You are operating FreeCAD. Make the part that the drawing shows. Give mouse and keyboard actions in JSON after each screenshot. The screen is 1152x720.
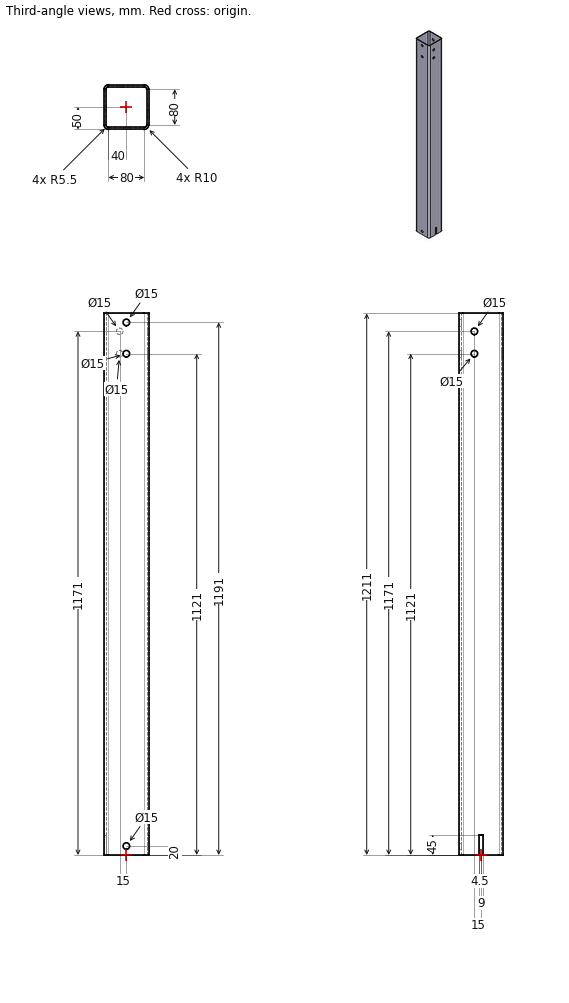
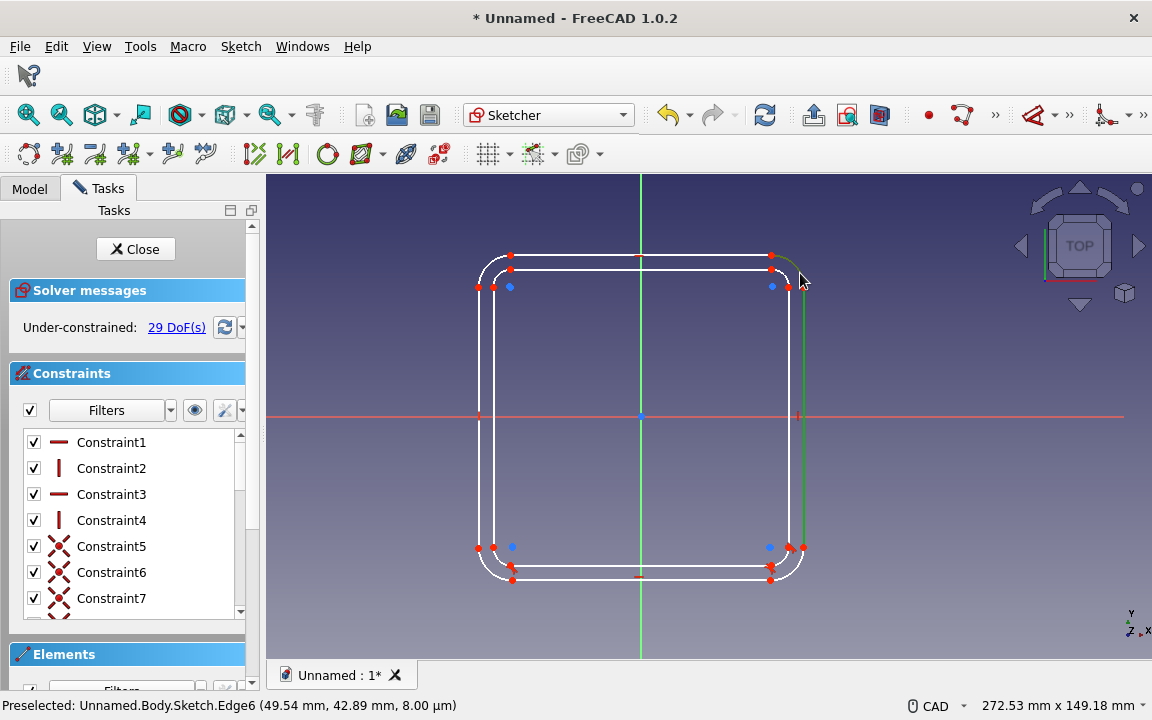
{"action": "key", "text": "t"}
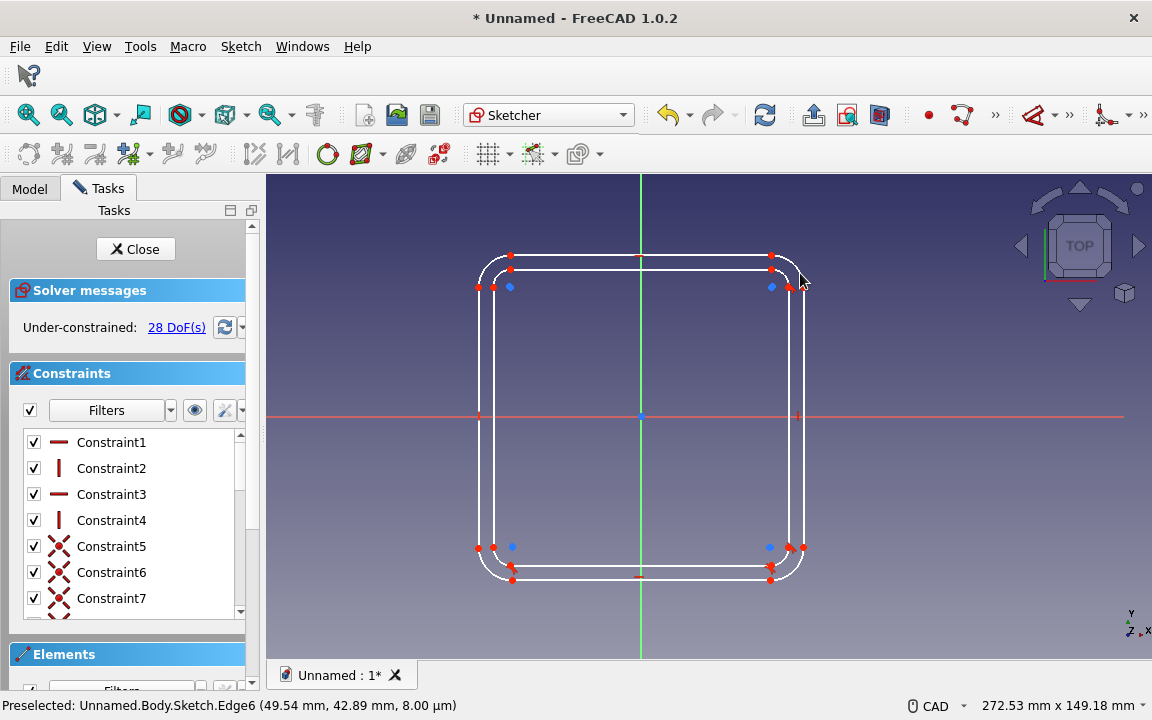
{"action": "left_click", "coordinate": [693, 255]}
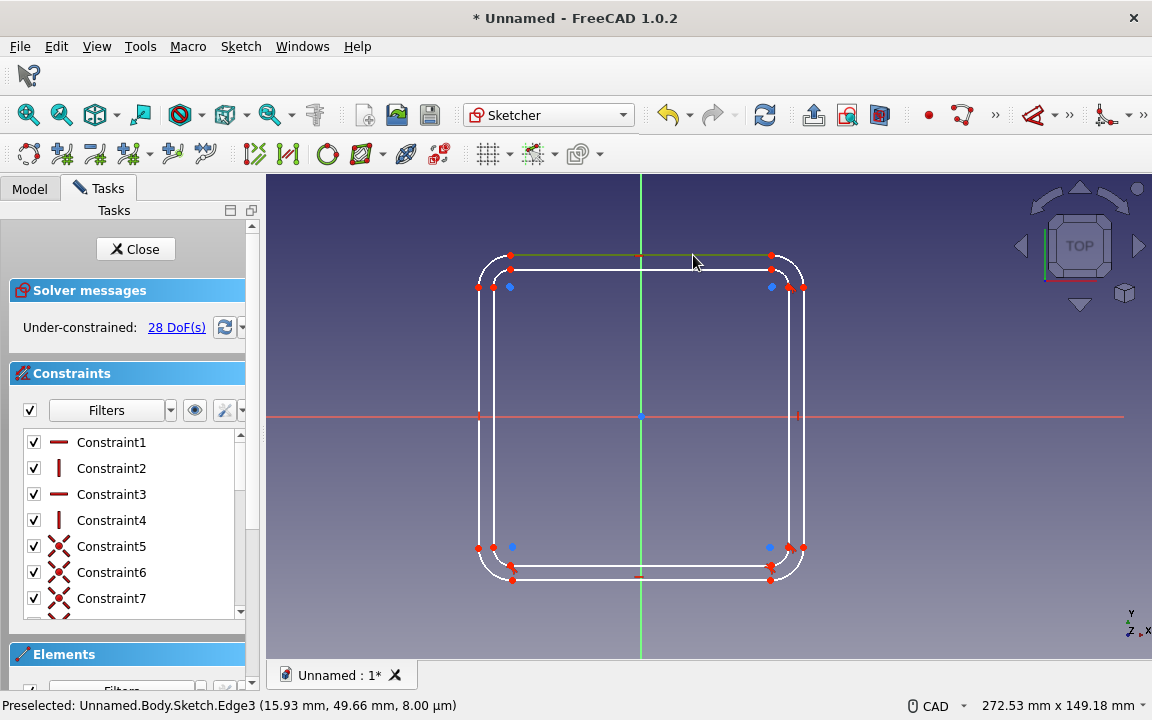
{"action": "left_click", "coordinate": [800, 273]}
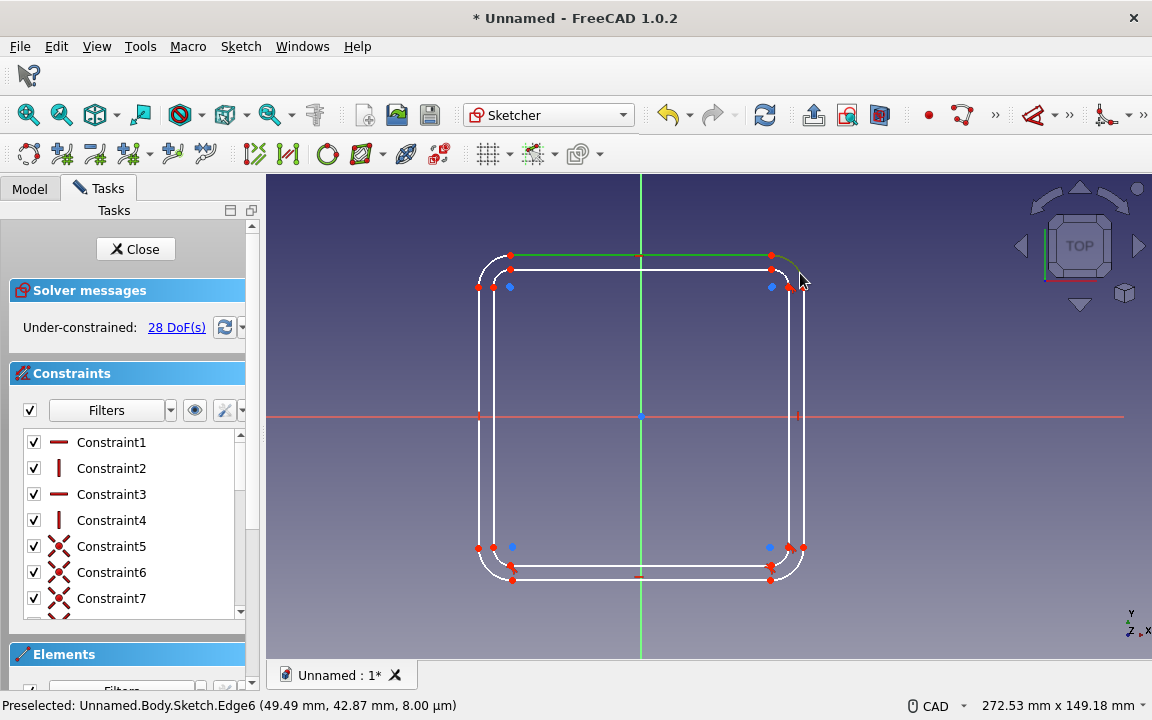
{"action": "key", "text": "t"}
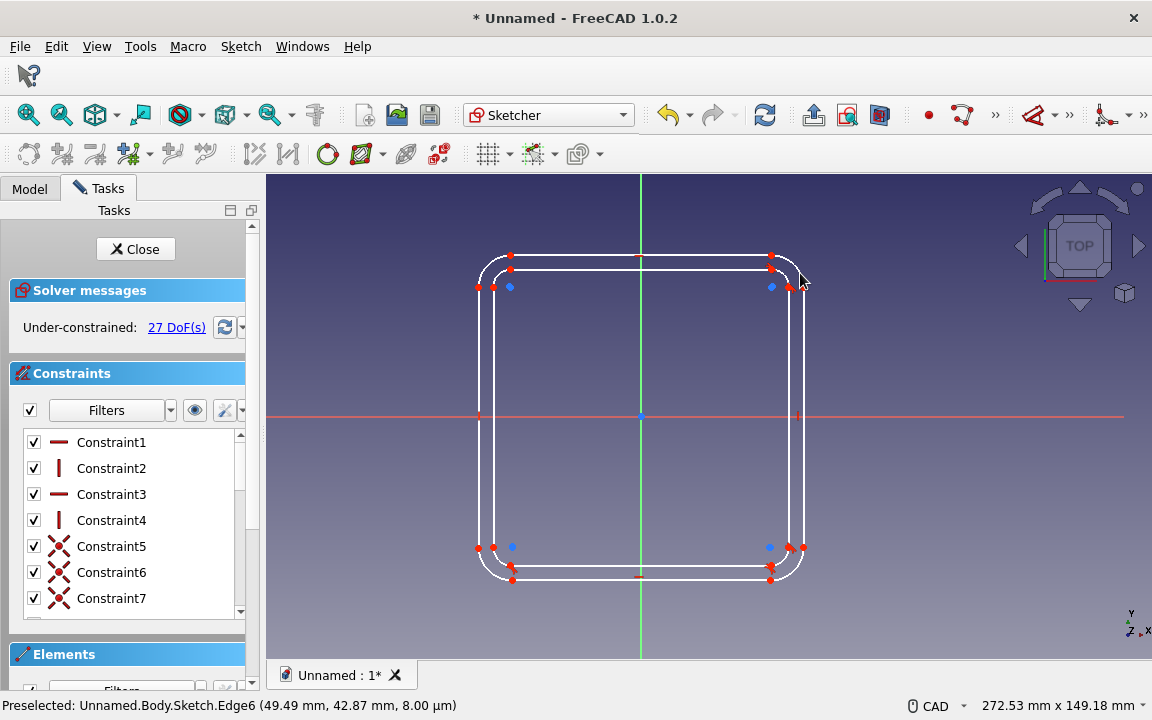
{"action": "left_click", "coordinate": [693, 255]}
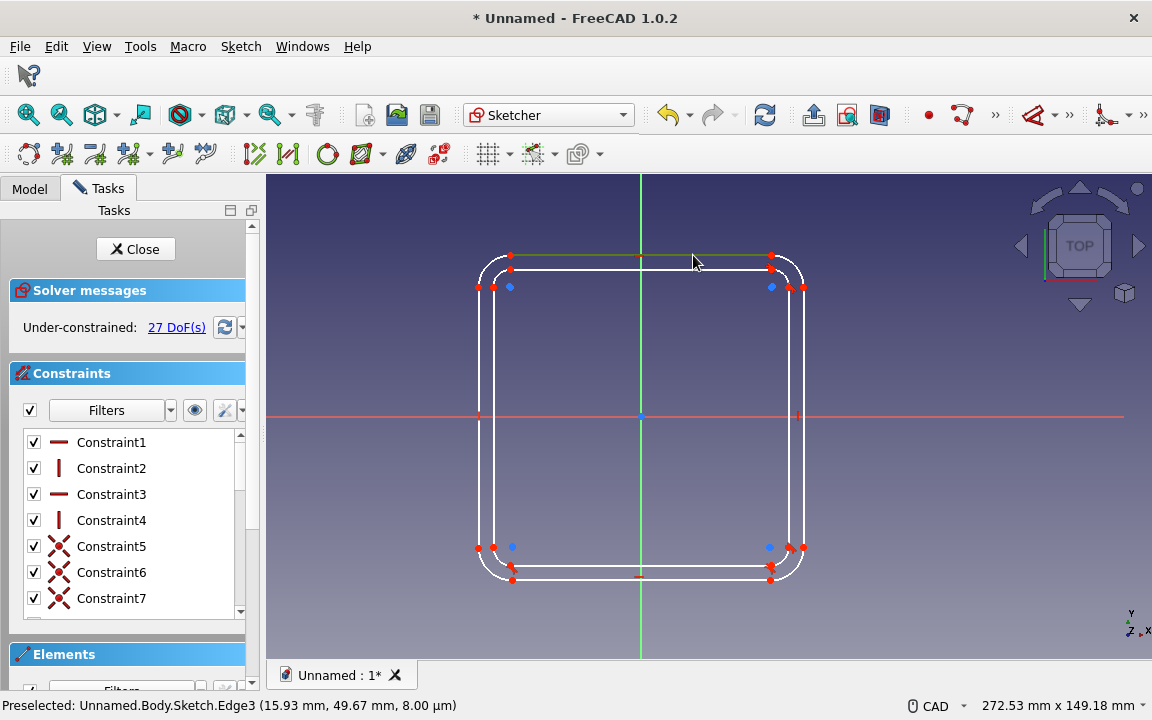
{"action": "left_click", "coordinate": [496, 259]}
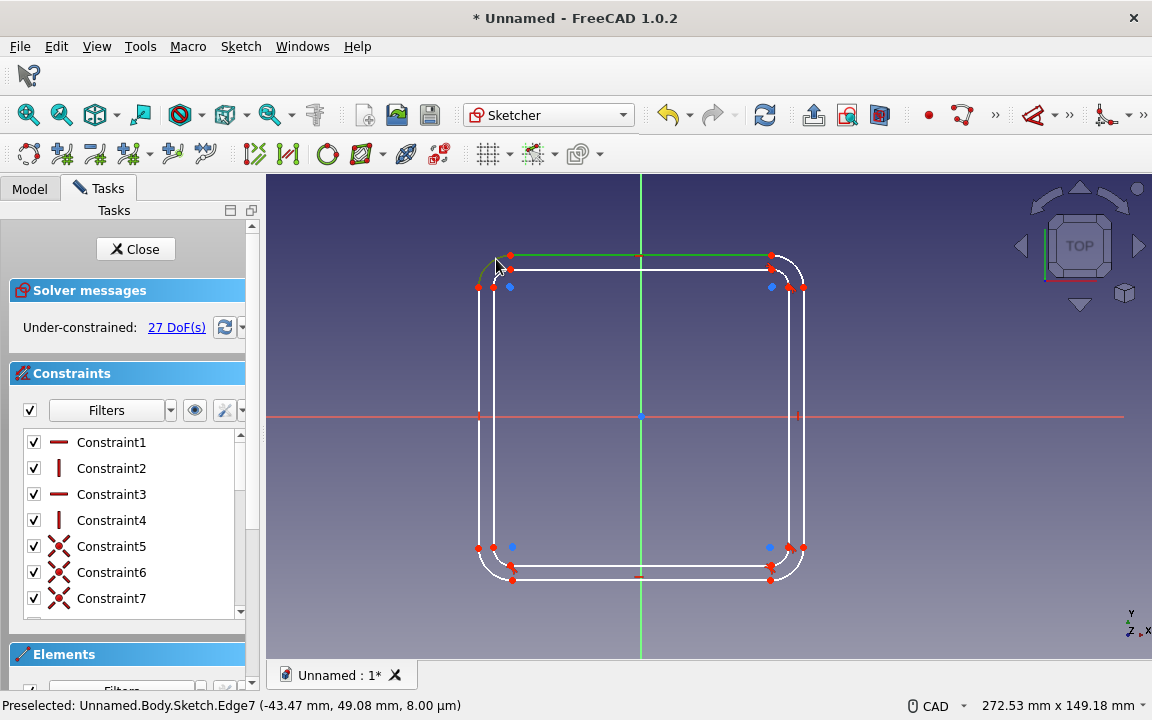
{"action": "key", "text": "t"}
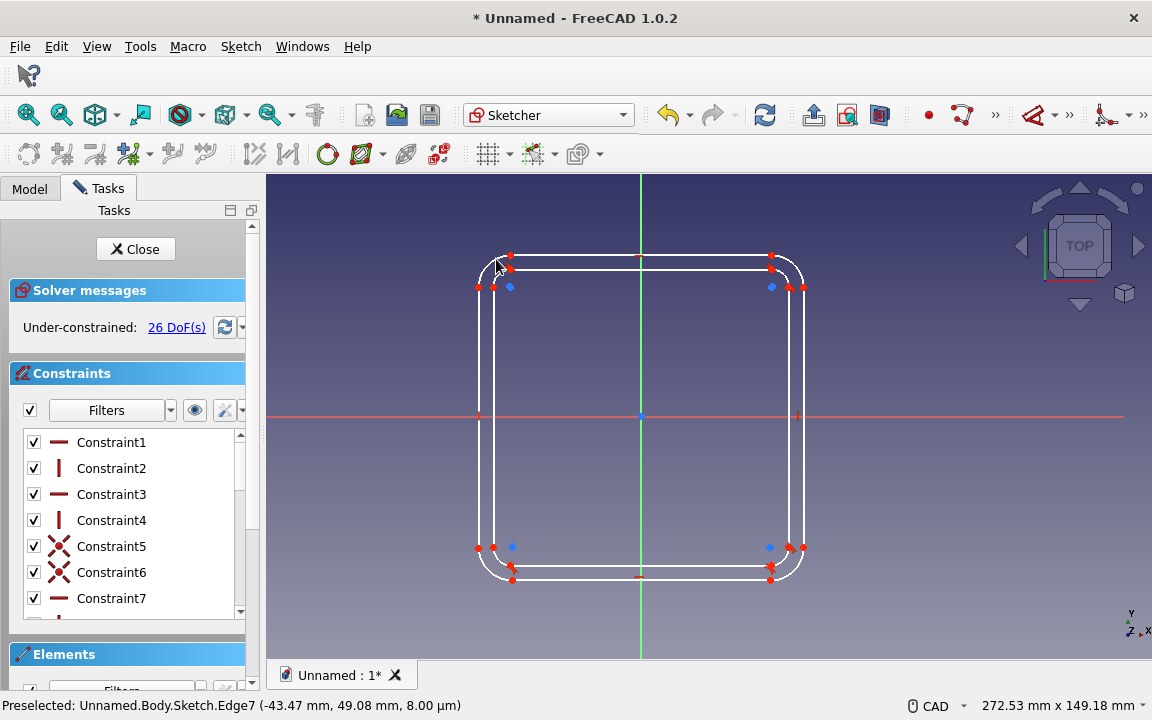
{"action": "left_click", "coordinate": [479, 366]}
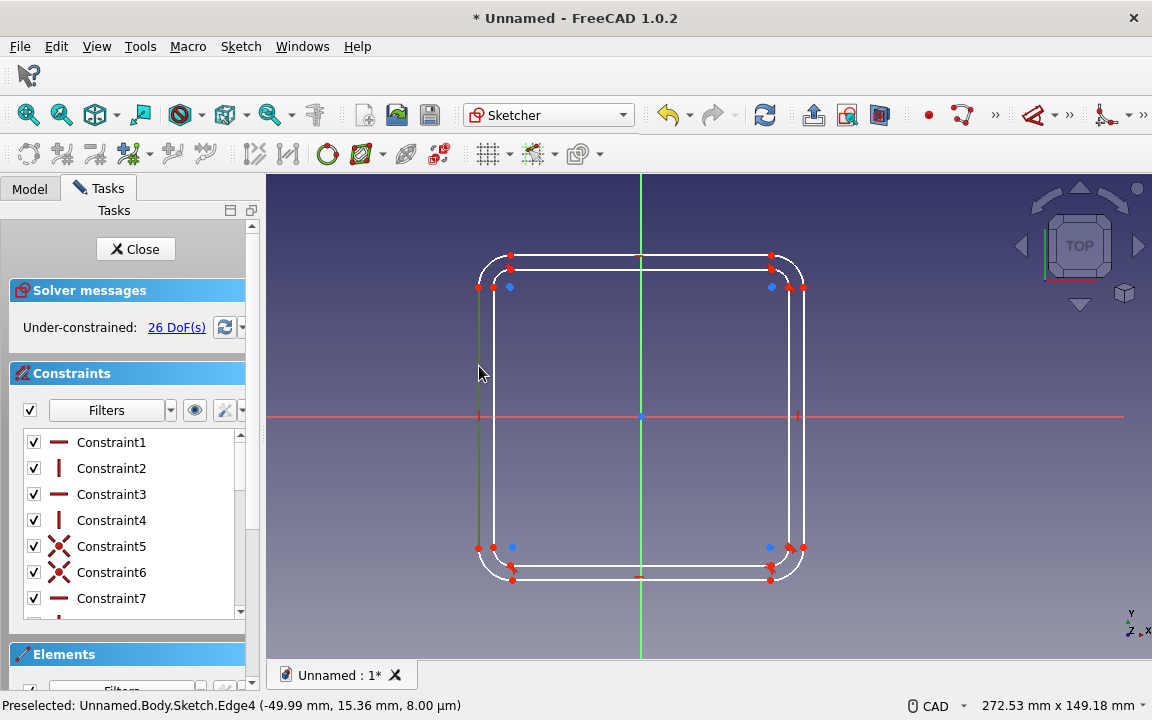
{"action": "left_click", "coordinate": [496, 259]}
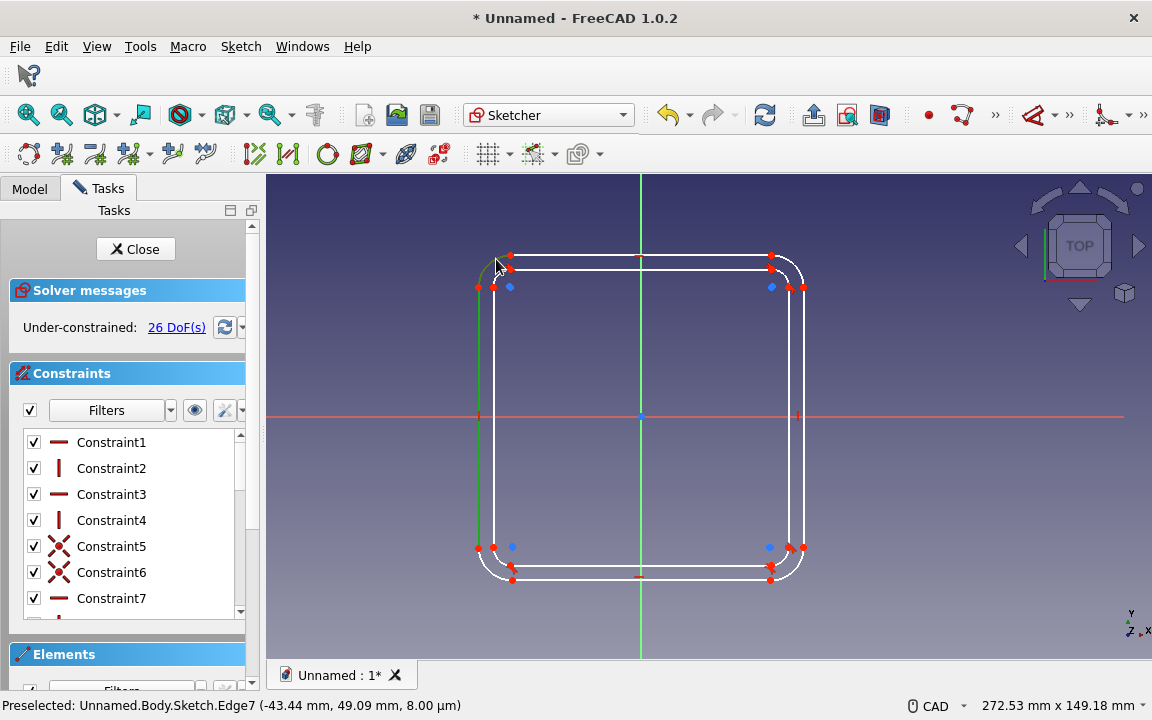
{"action": "key", "text": "t"}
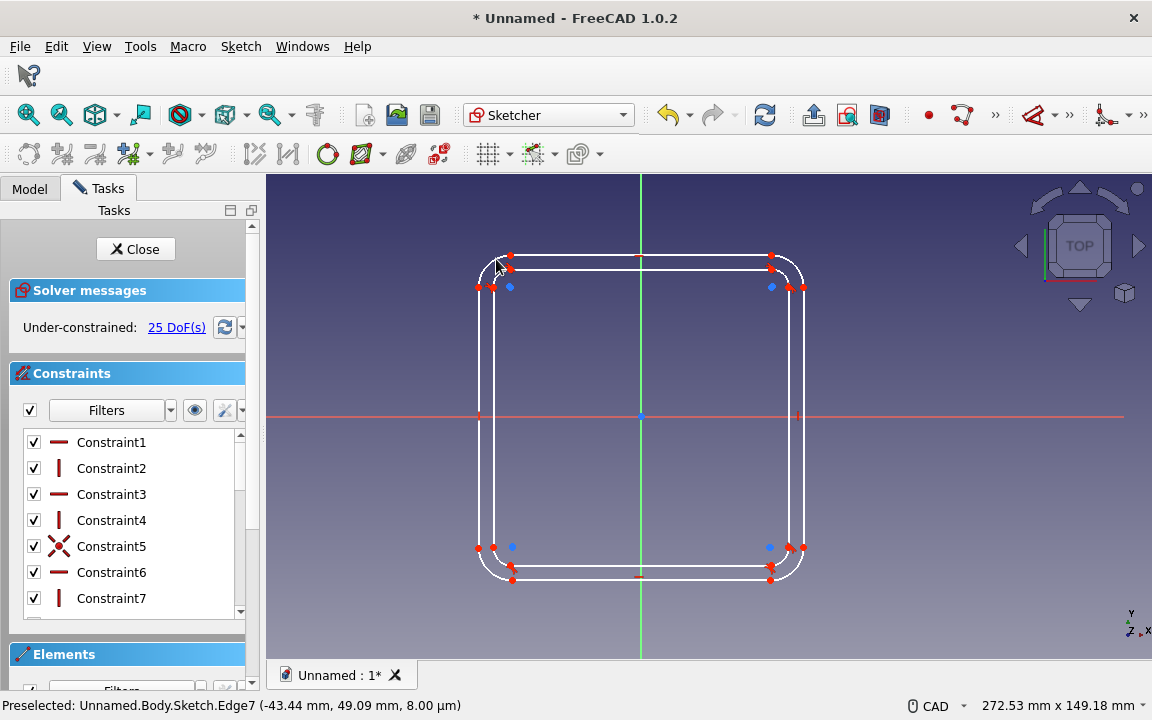
{"action": "left_click", "coordinate": [479, 366]}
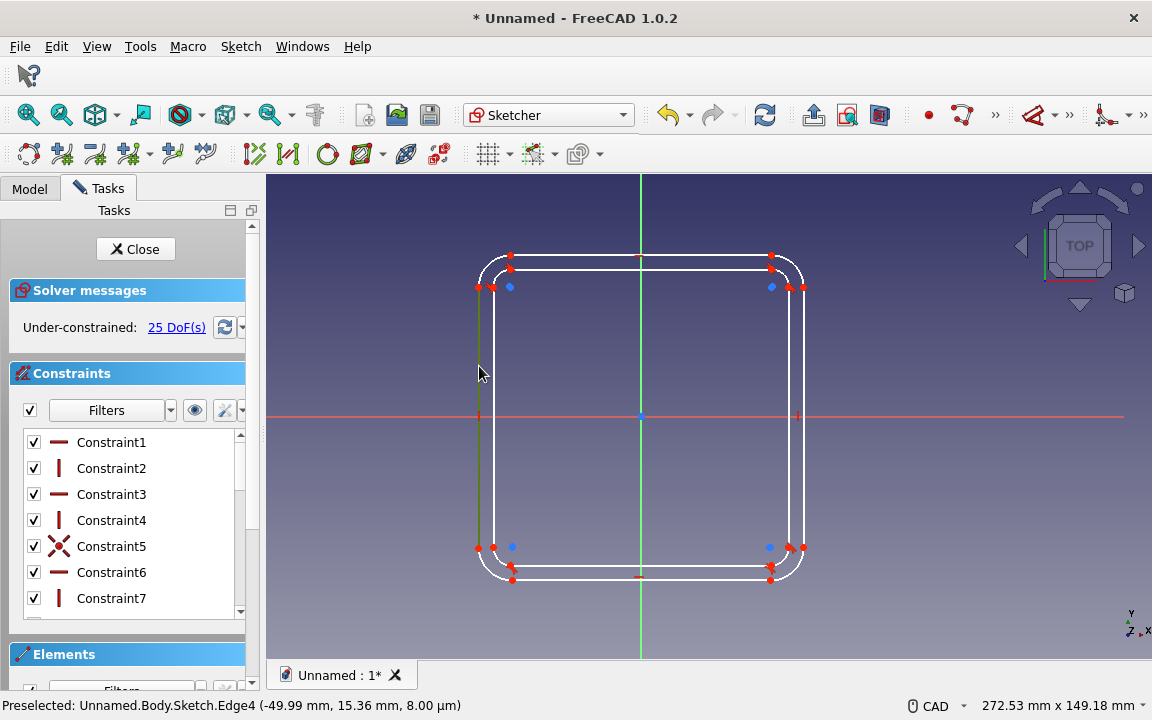
{"action": "left_click", "coordinate": [483, 563]}